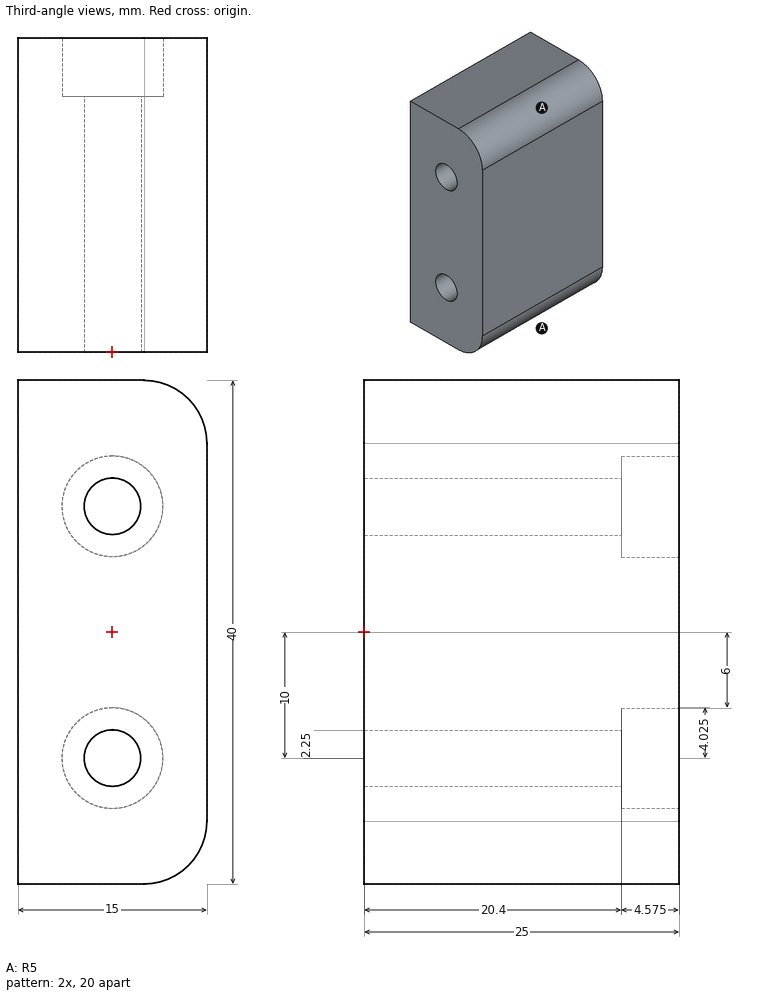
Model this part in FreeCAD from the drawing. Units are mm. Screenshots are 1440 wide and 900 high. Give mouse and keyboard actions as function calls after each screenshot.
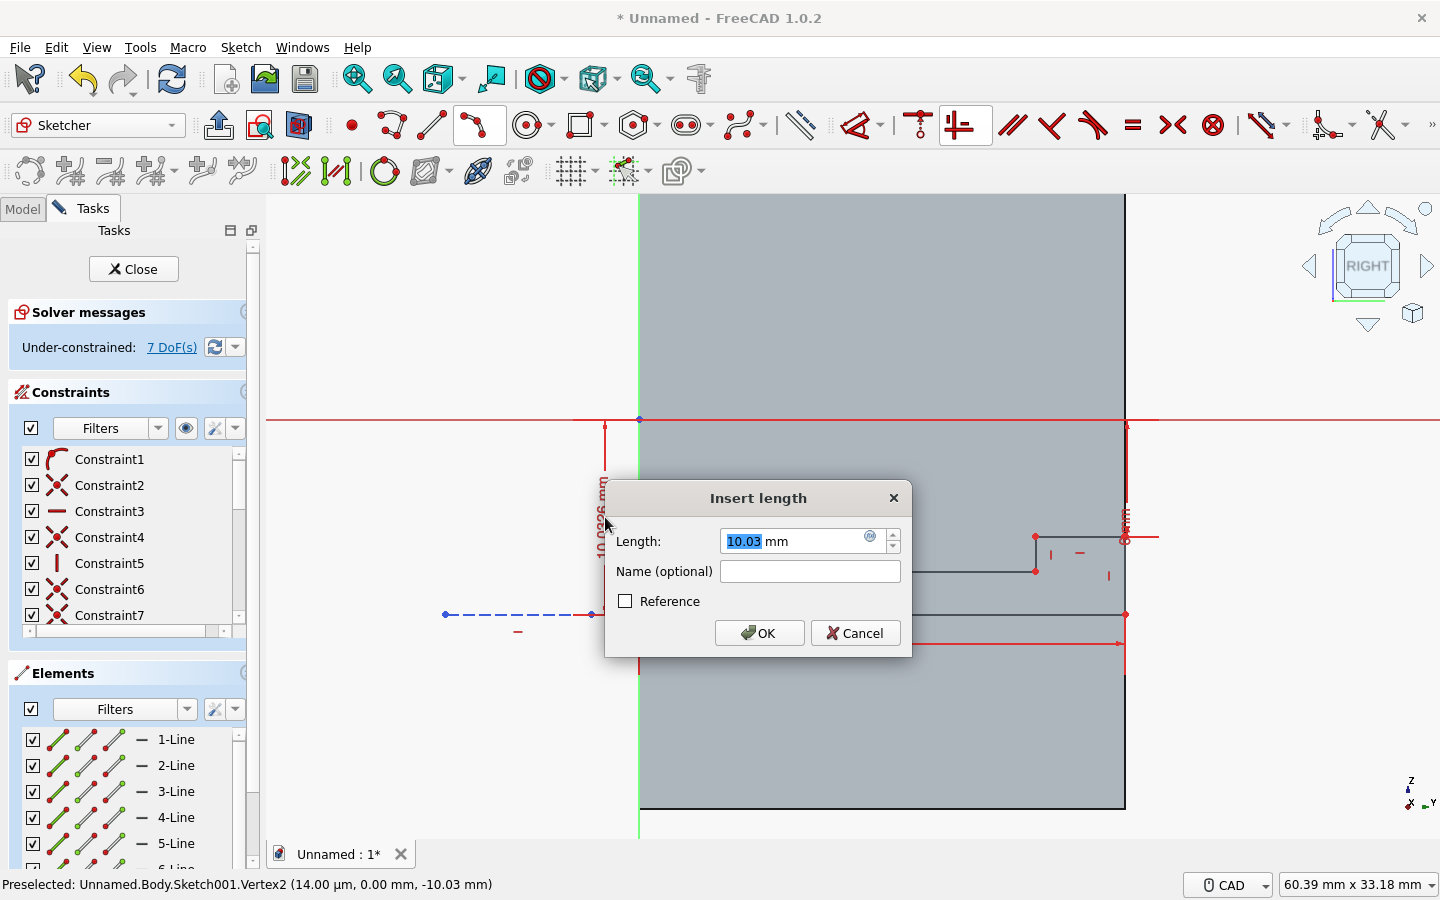
text(10)
key(Return)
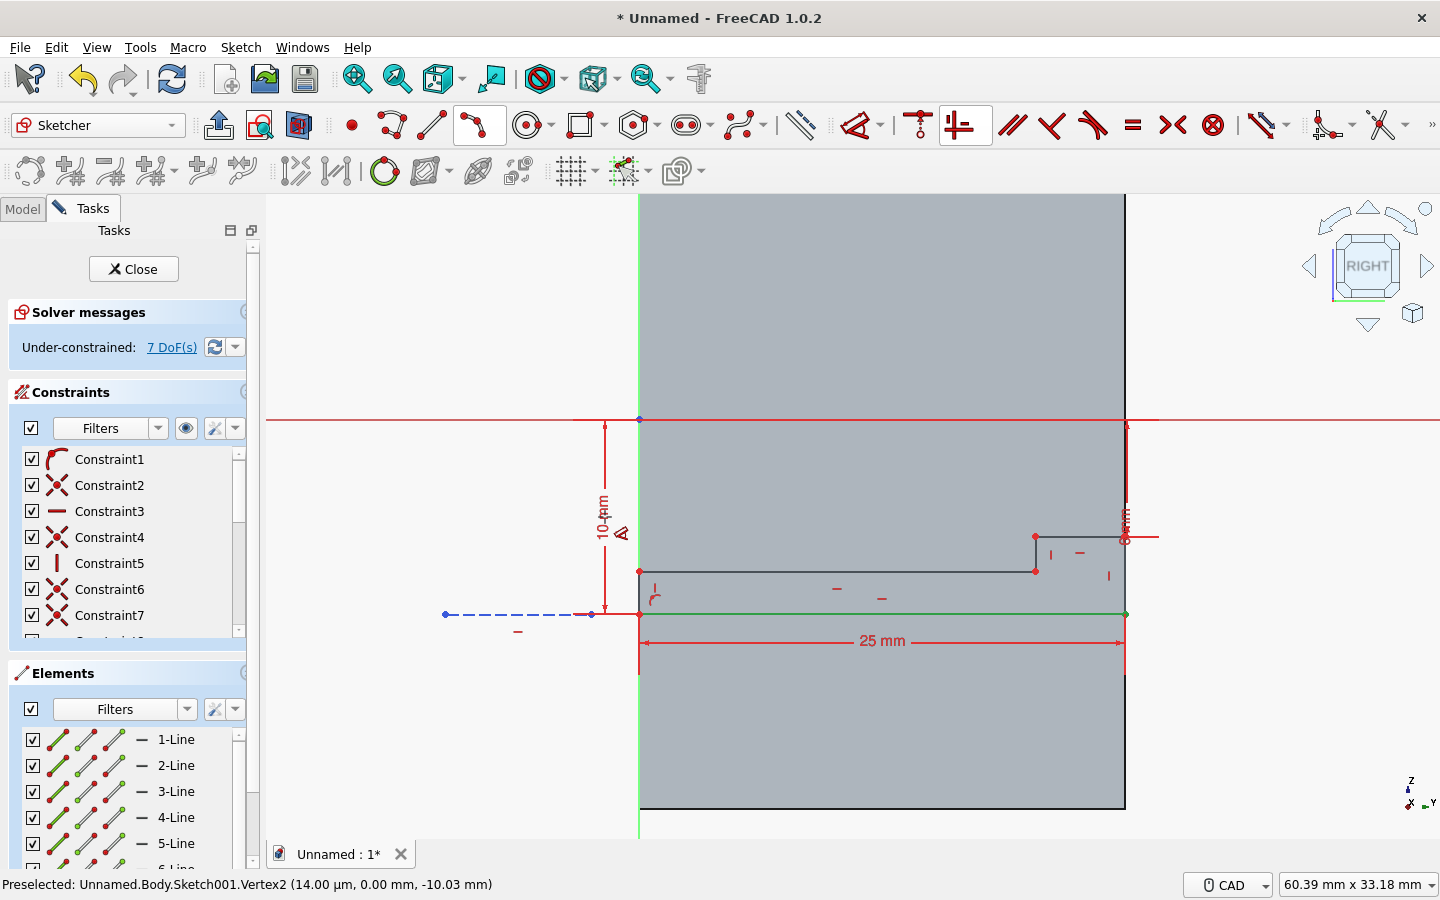
click(591, 615)
click(557, 473)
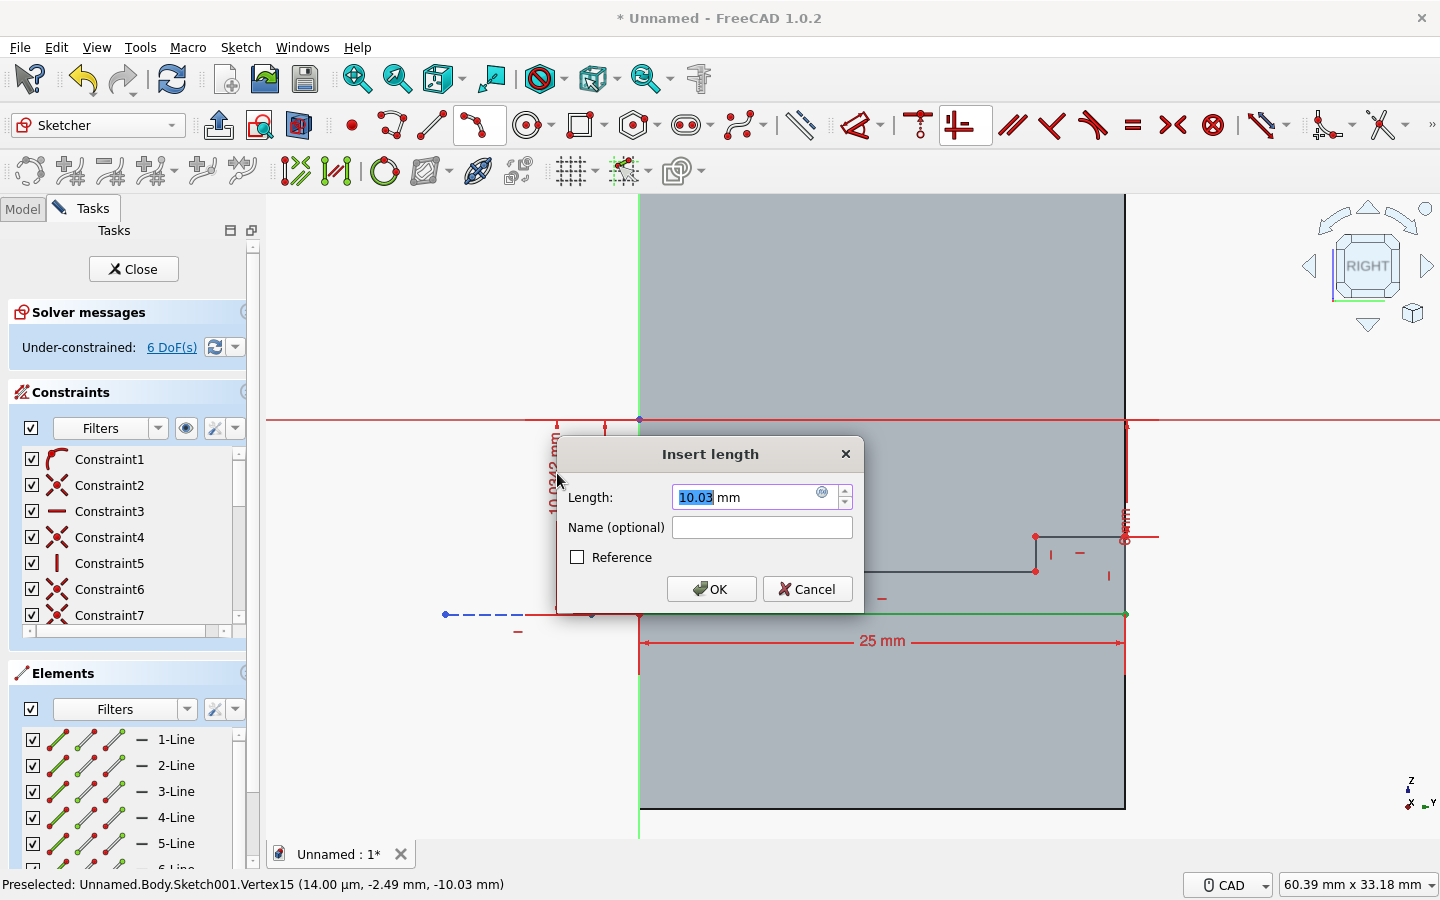
text(10)
key(Return)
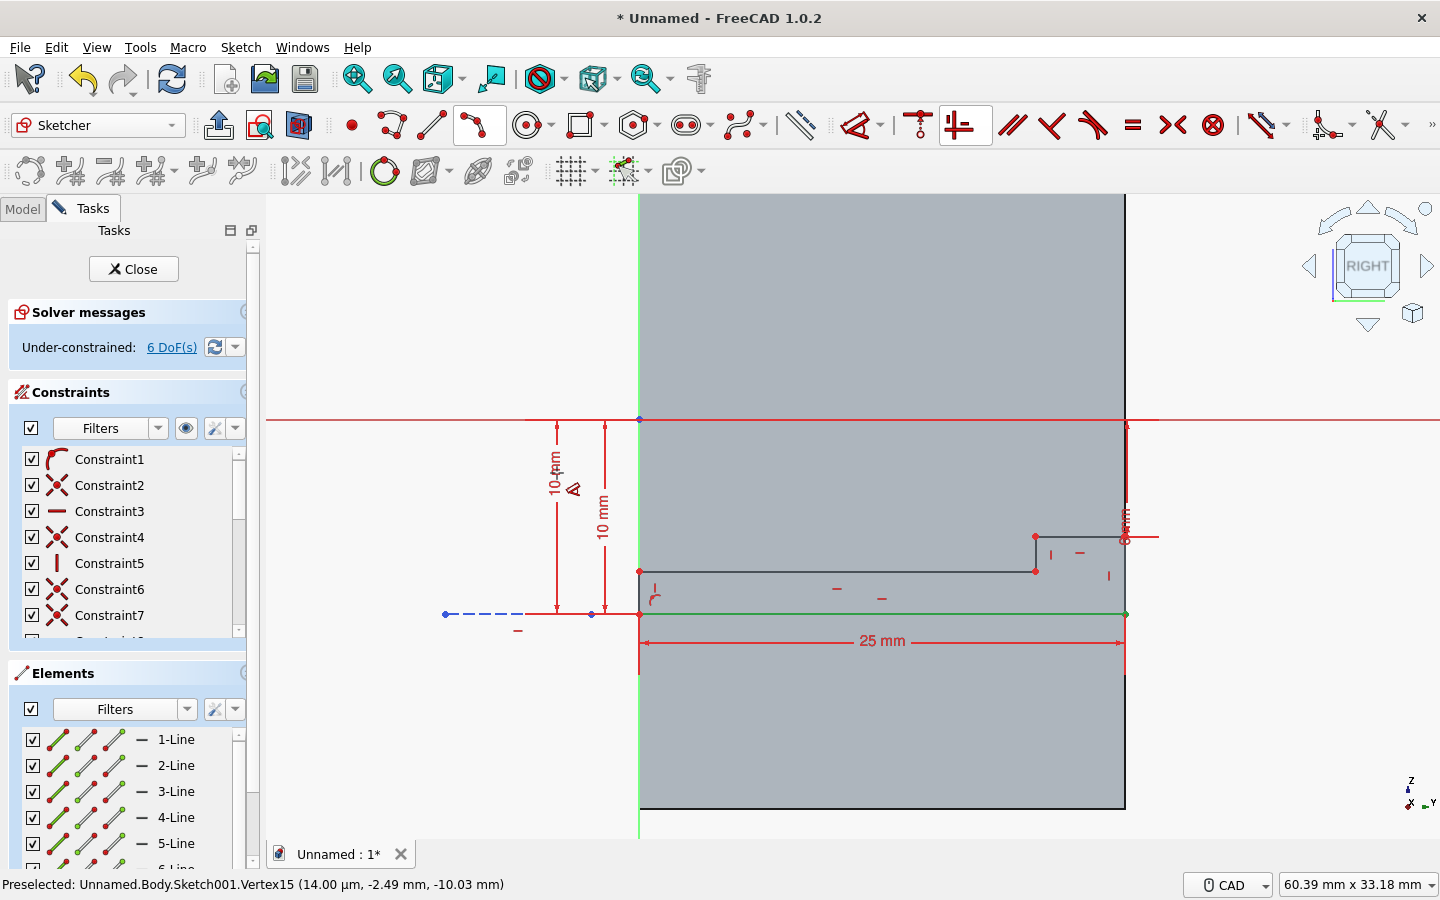
click(639, 585)
click(605, 593)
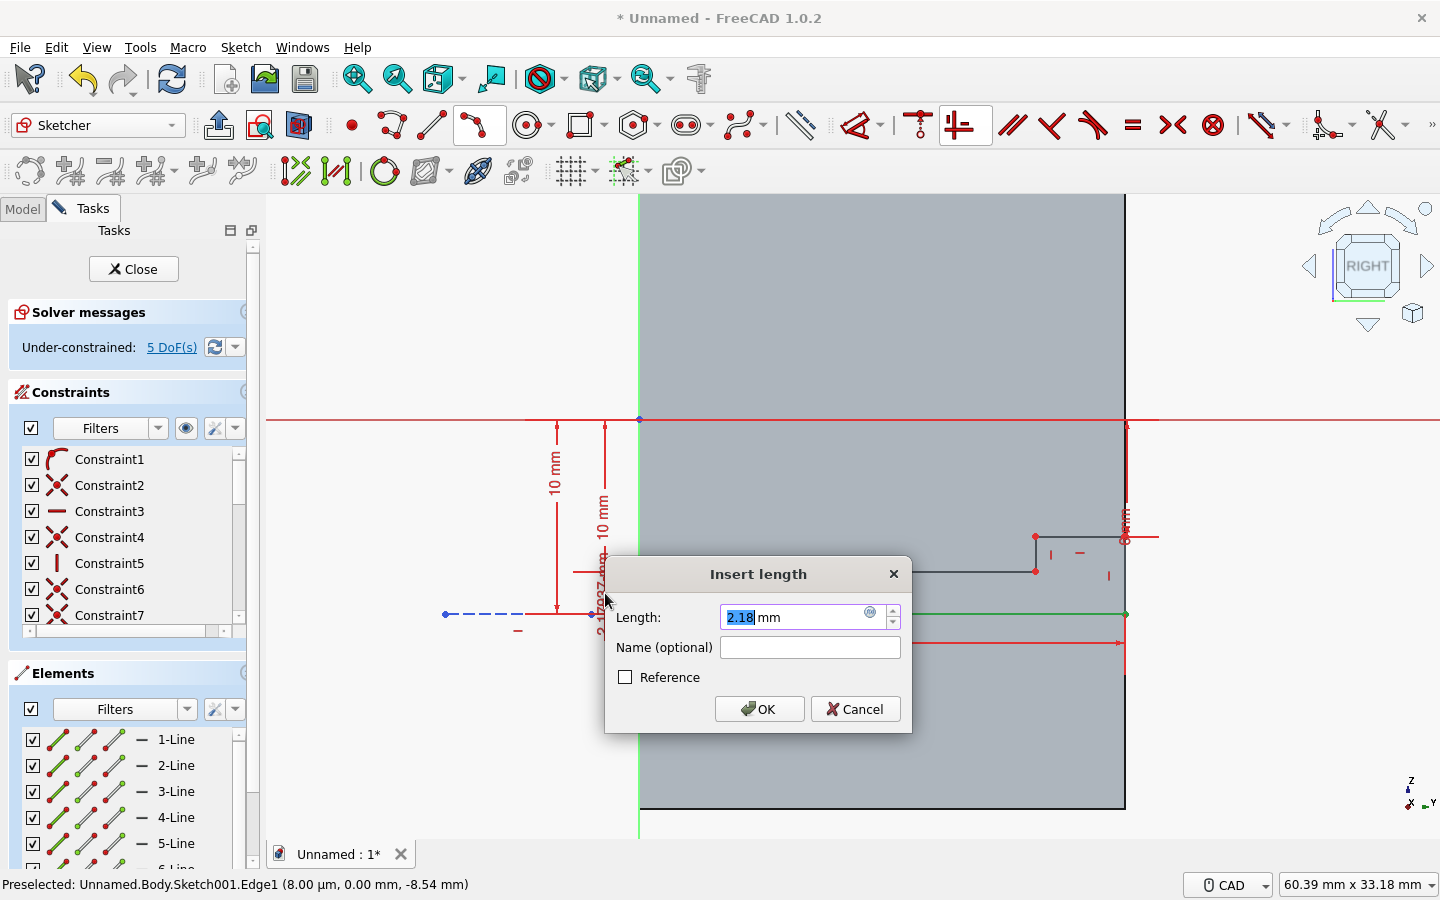
text(2.25)
key(Return)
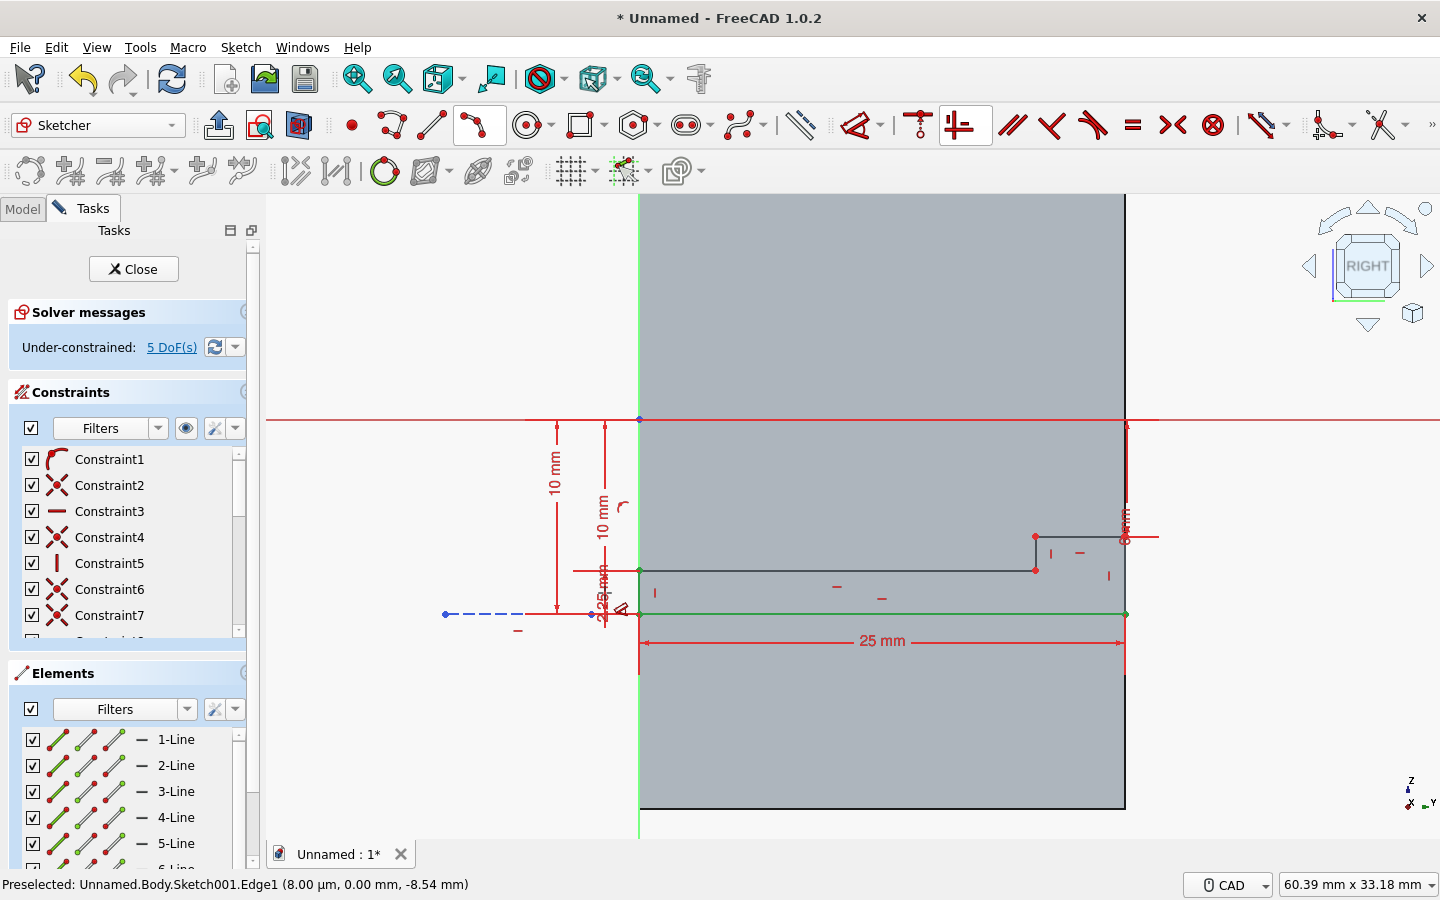
click(917, 571)
click(838, 537)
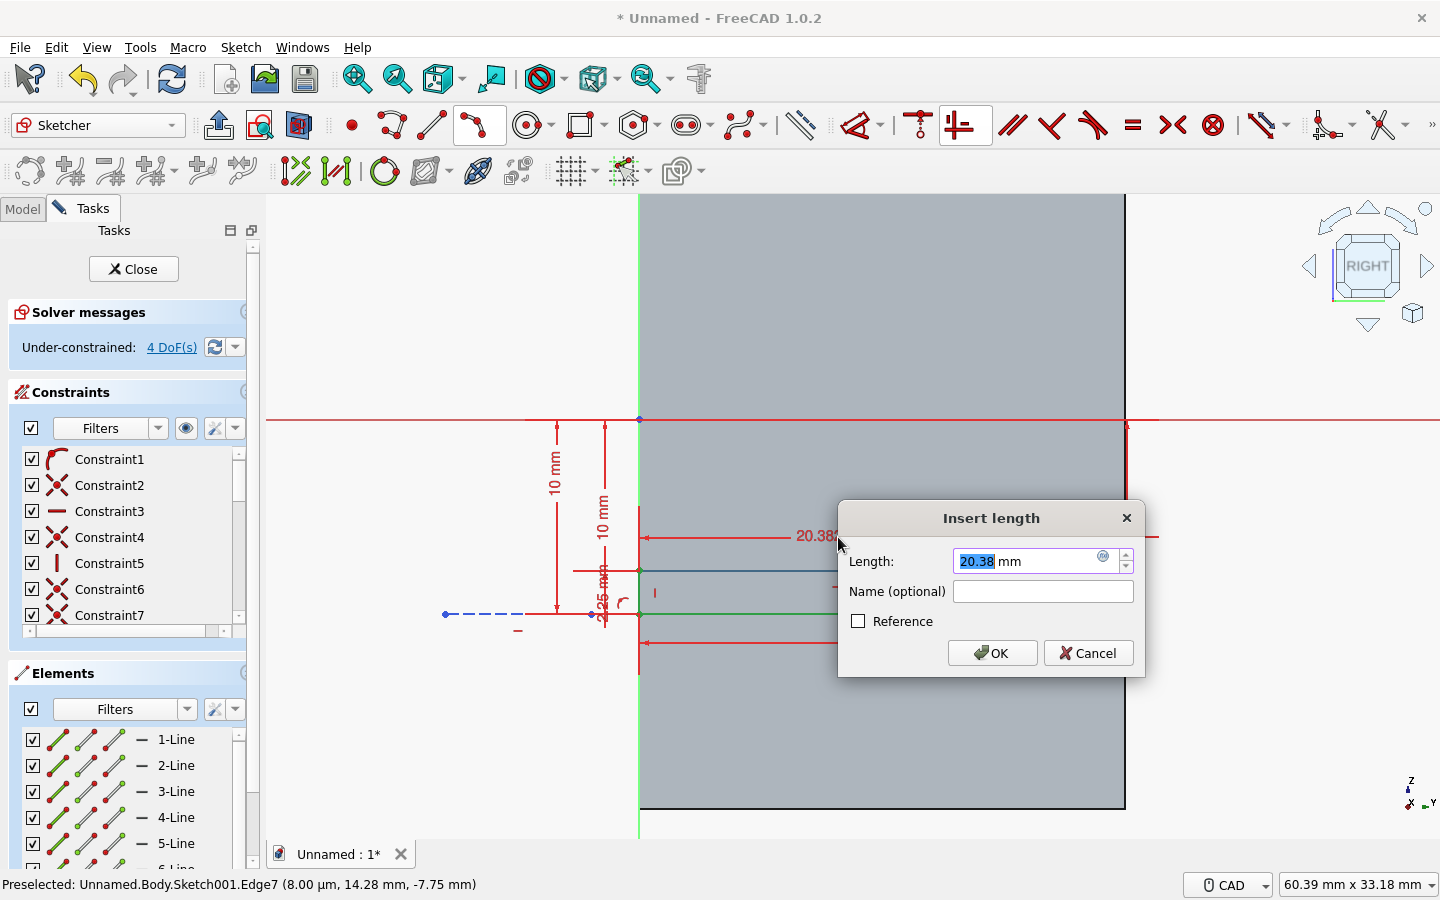
text(20.4)
key(Return)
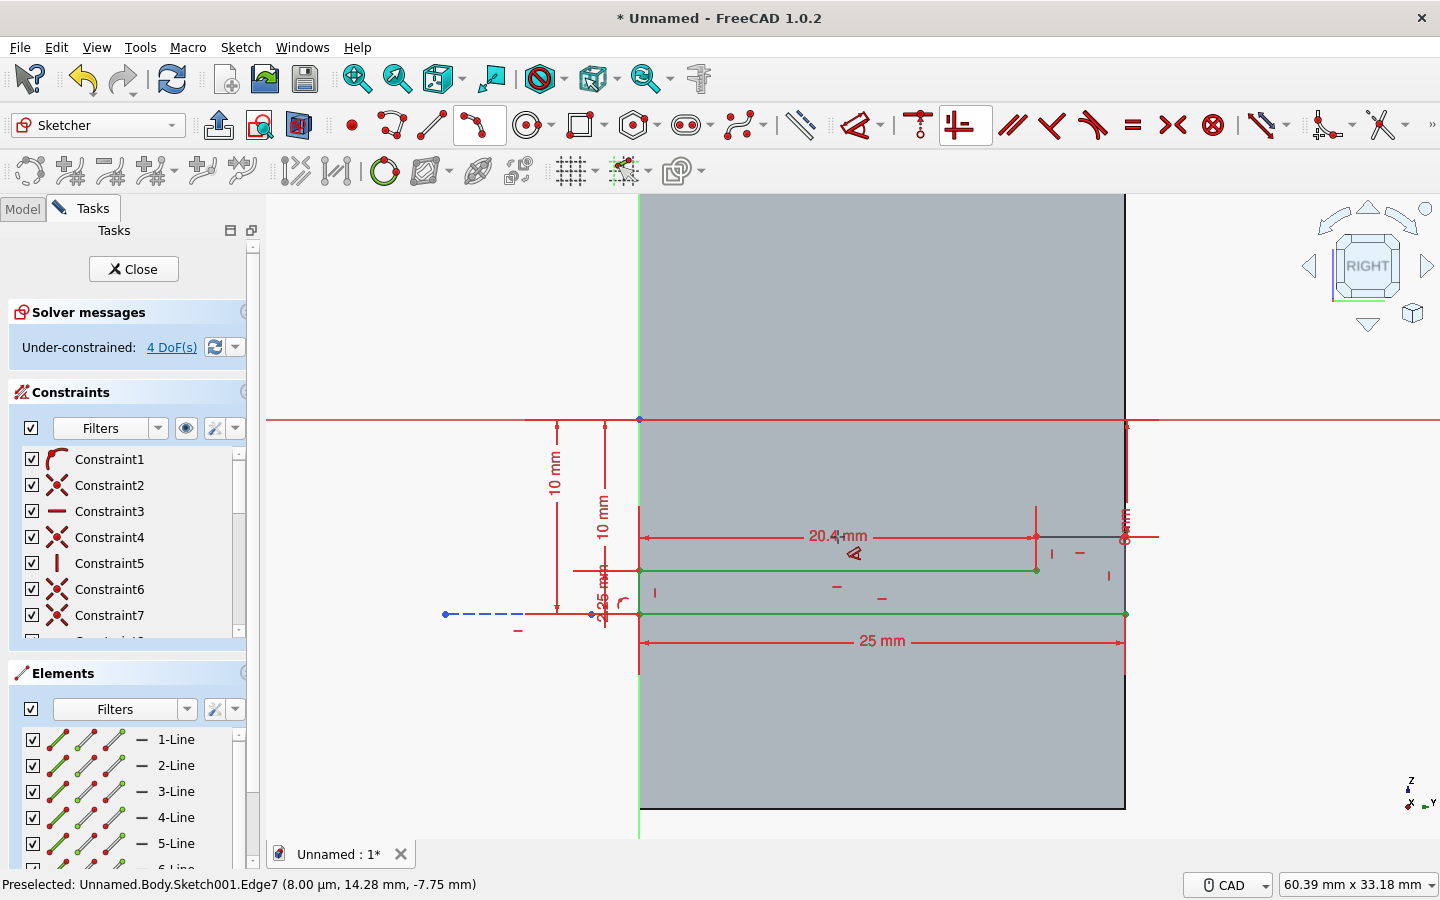
click(1125, 591)
click(1159, 576)